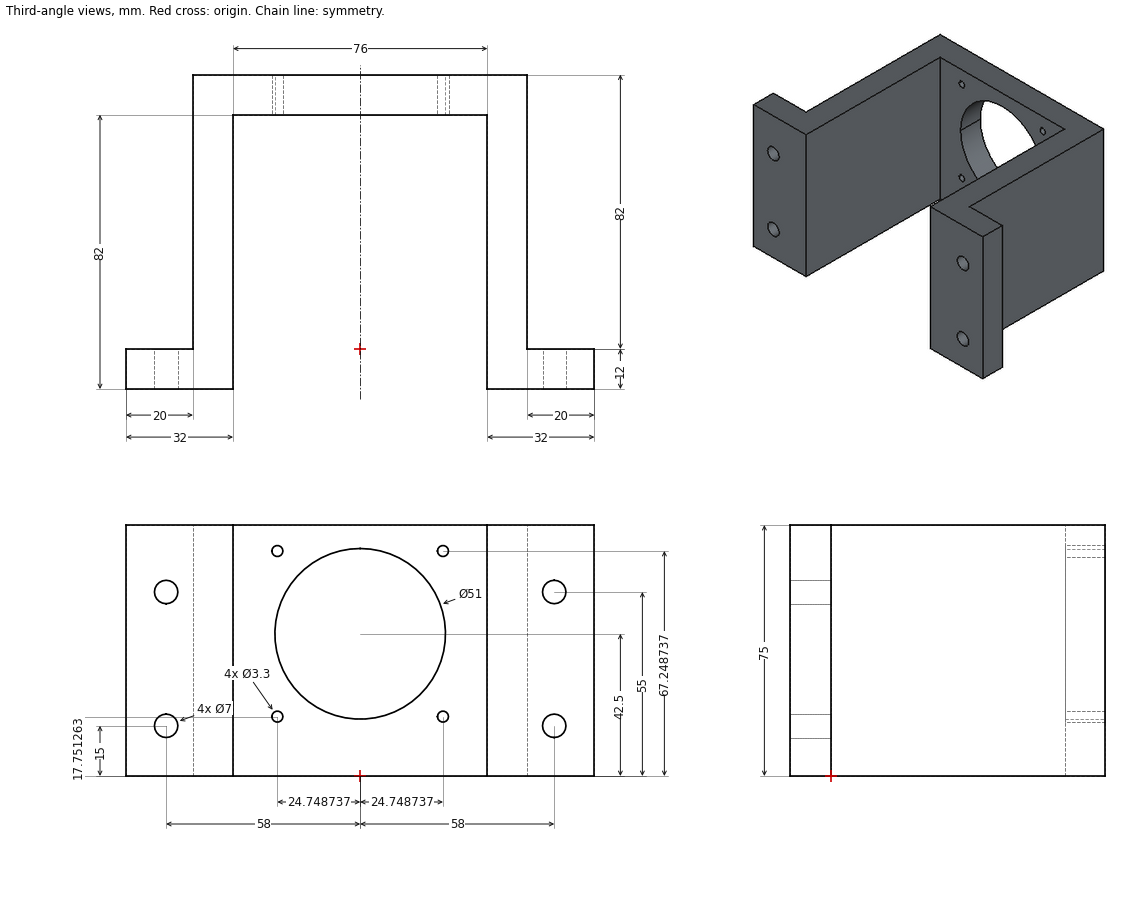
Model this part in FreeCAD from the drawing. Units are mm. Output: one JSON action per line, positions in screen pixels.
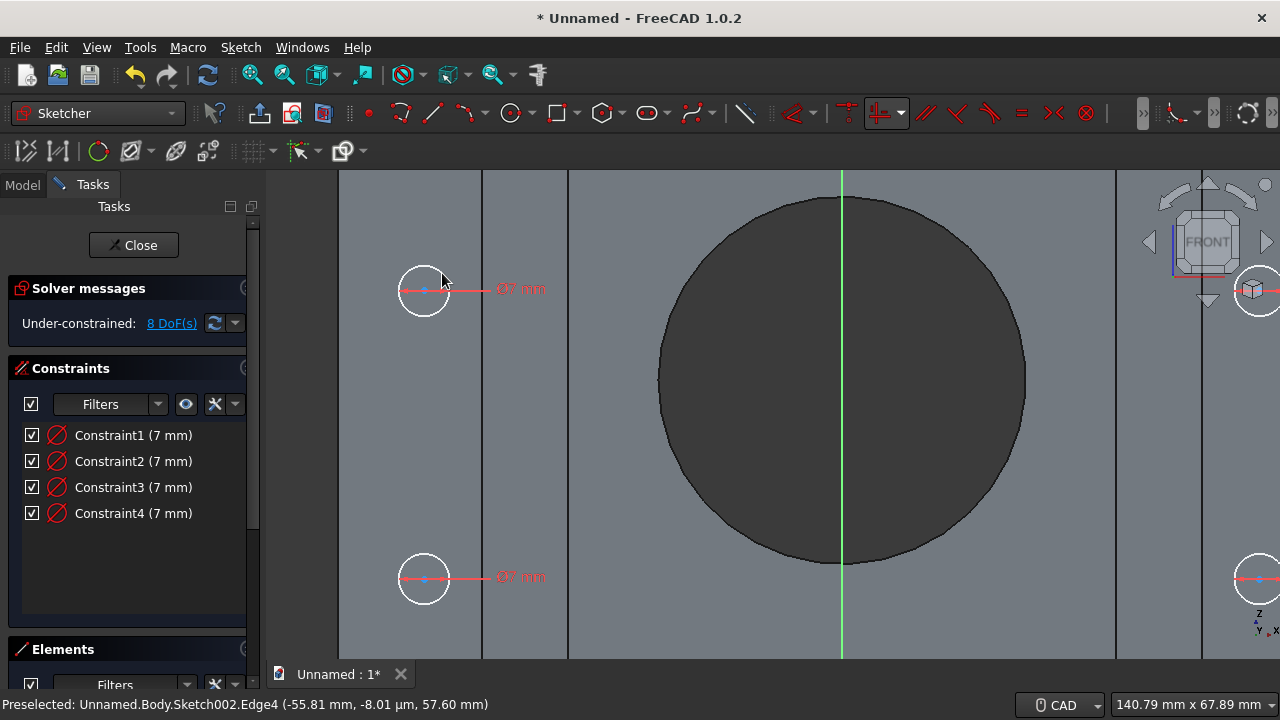
{"action": "left_click", "coordinate": [424, 579]}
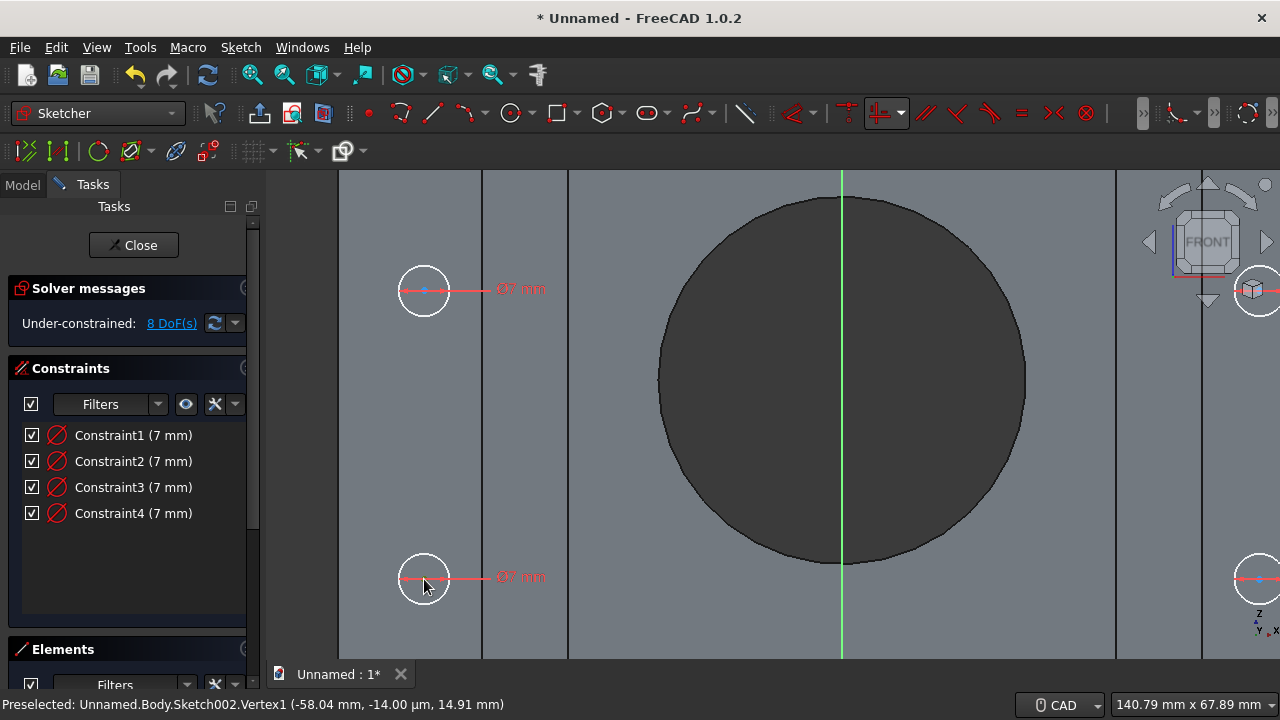
{"action": "scroll", "coordinate": [425, 290], "scroll_direction": "down", "scroll_amount": 2}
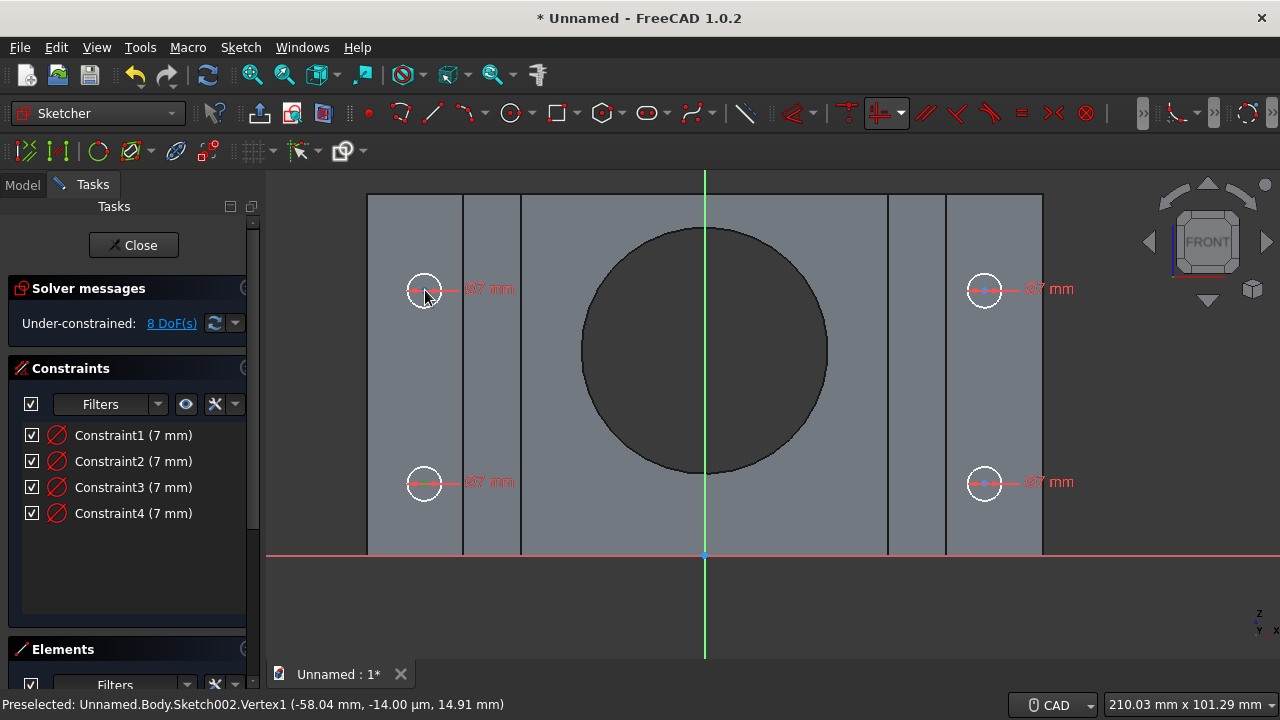
{"action": "left_click", "coordinate": [985, 484]}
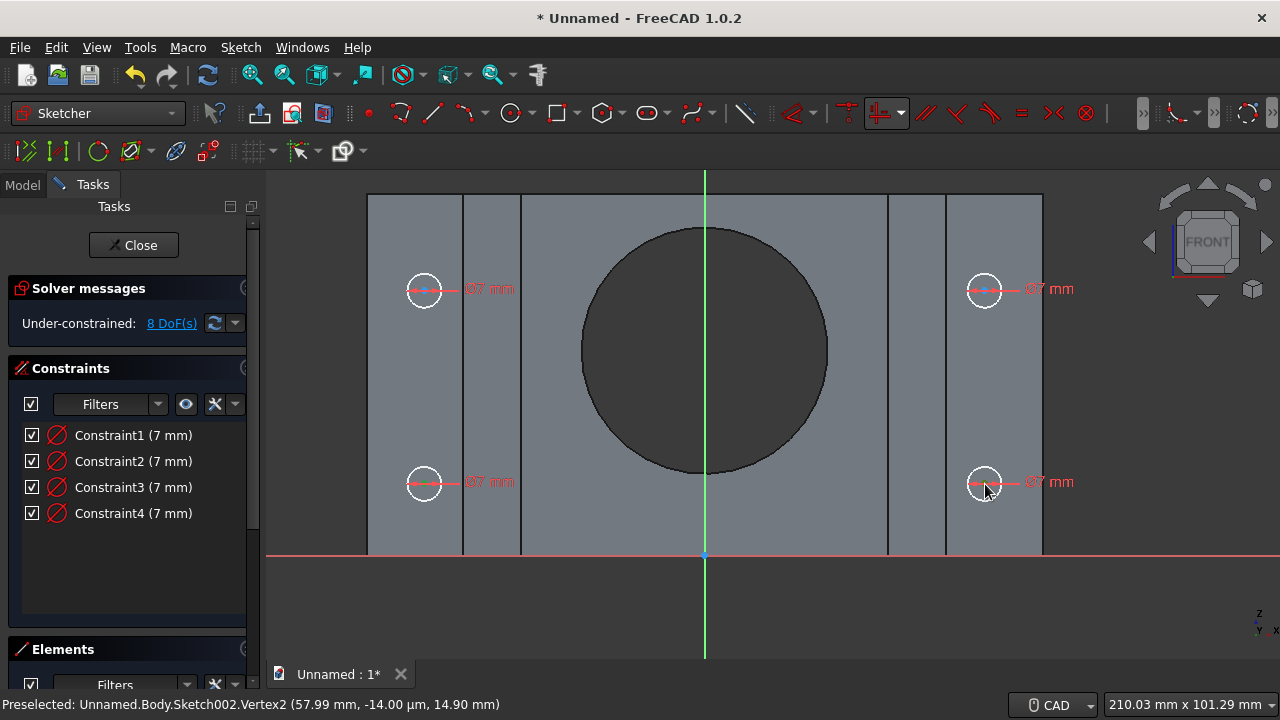
{"action": "key", "text": "h"}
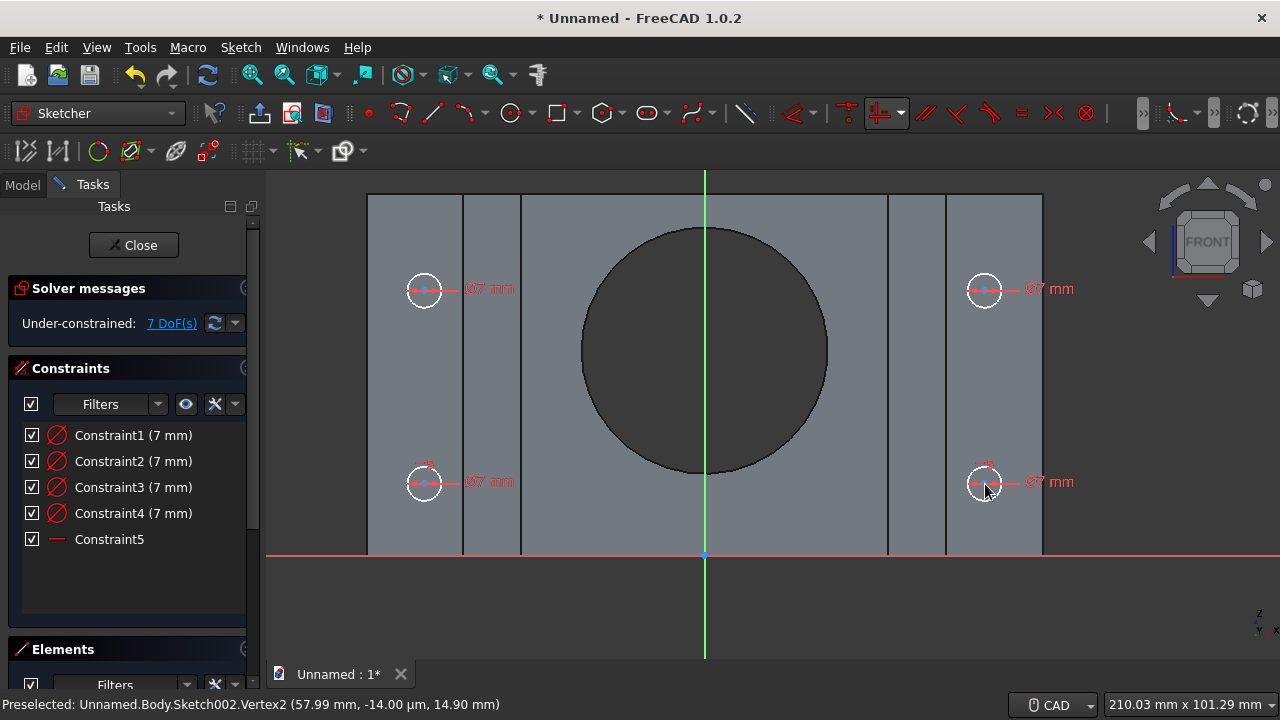
{"action": "left_click", "coordinate": [985, 484]}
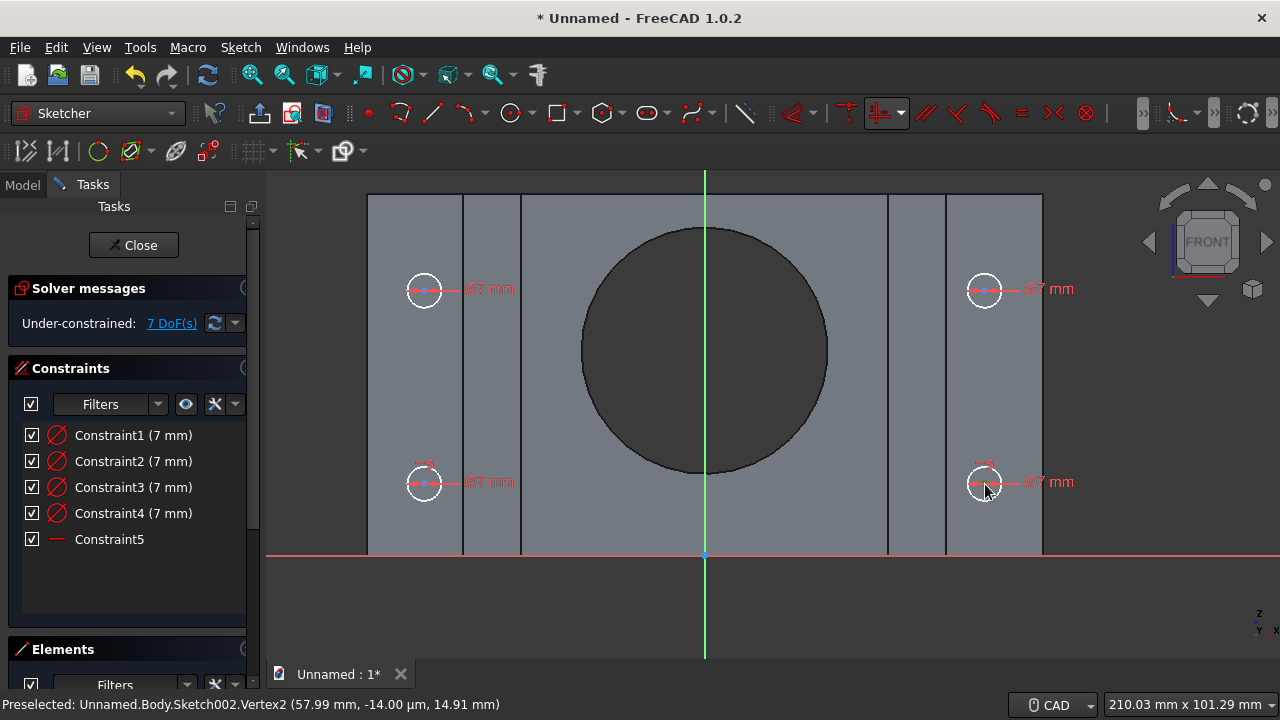
{"action": "left_click", "coordinate": [985, 291]}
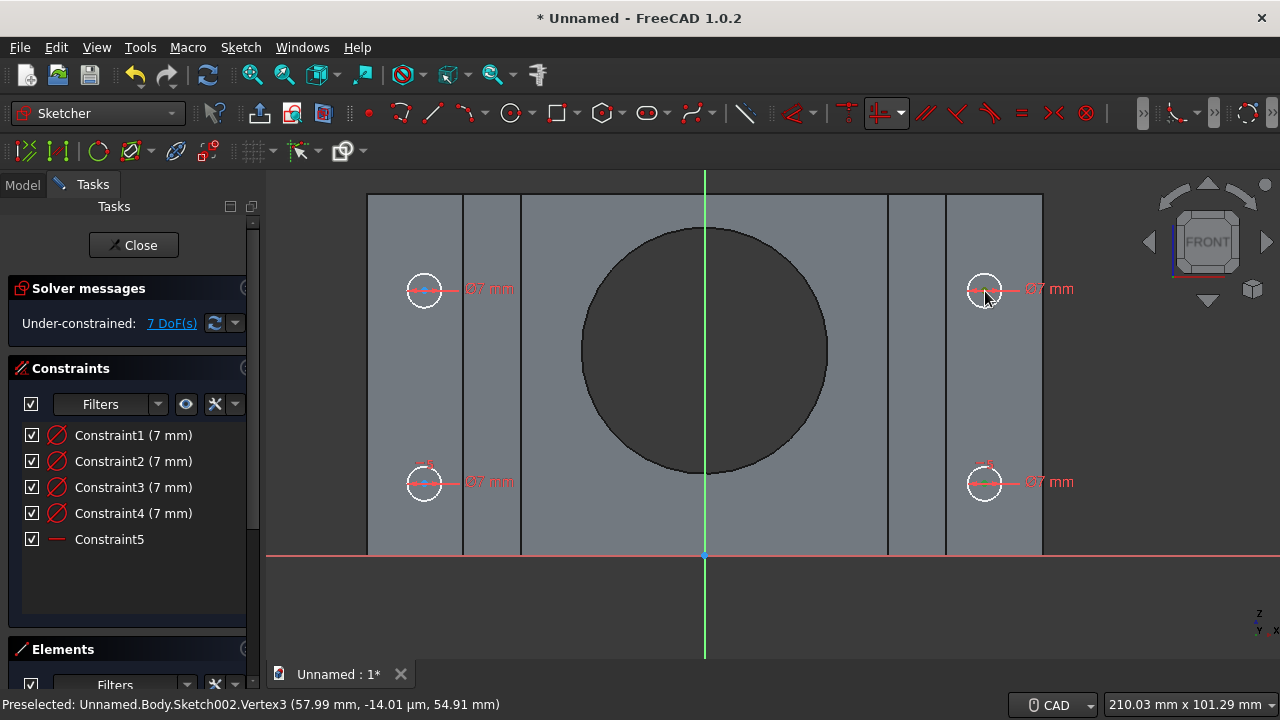
{"action": "key", "text": "v"}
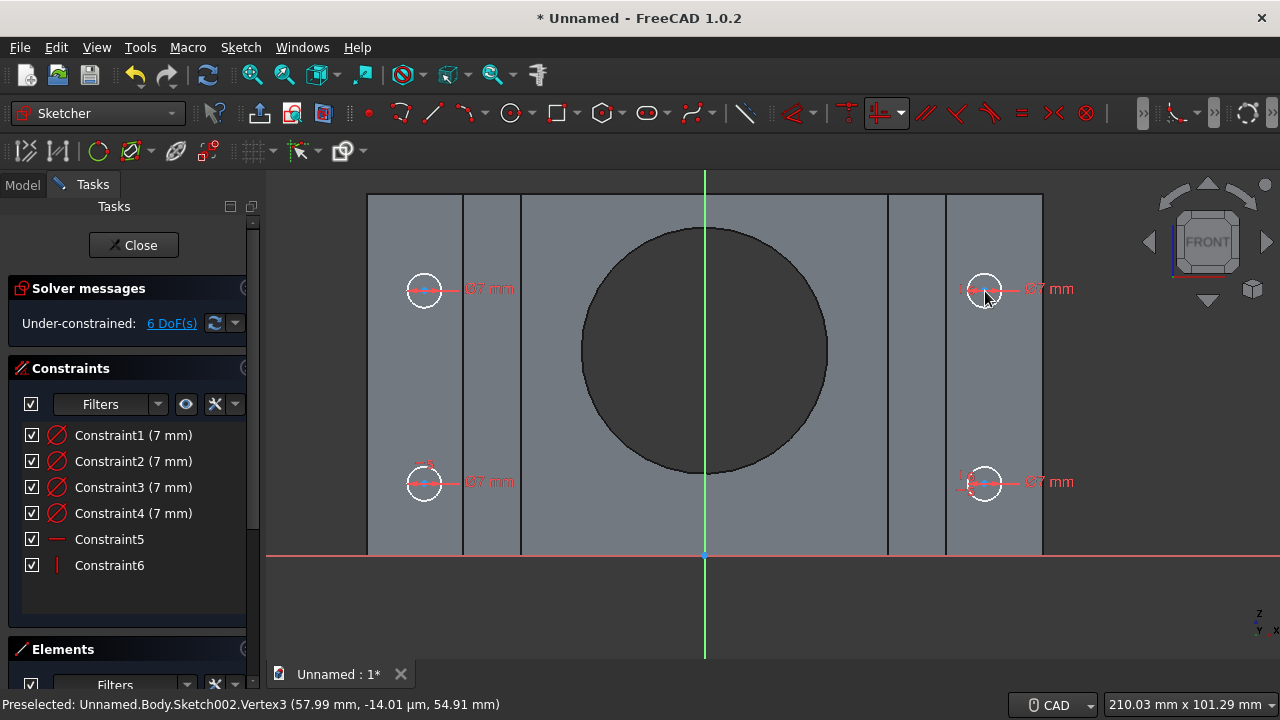
{"action": "left_click", "coordinate": [424, 484]}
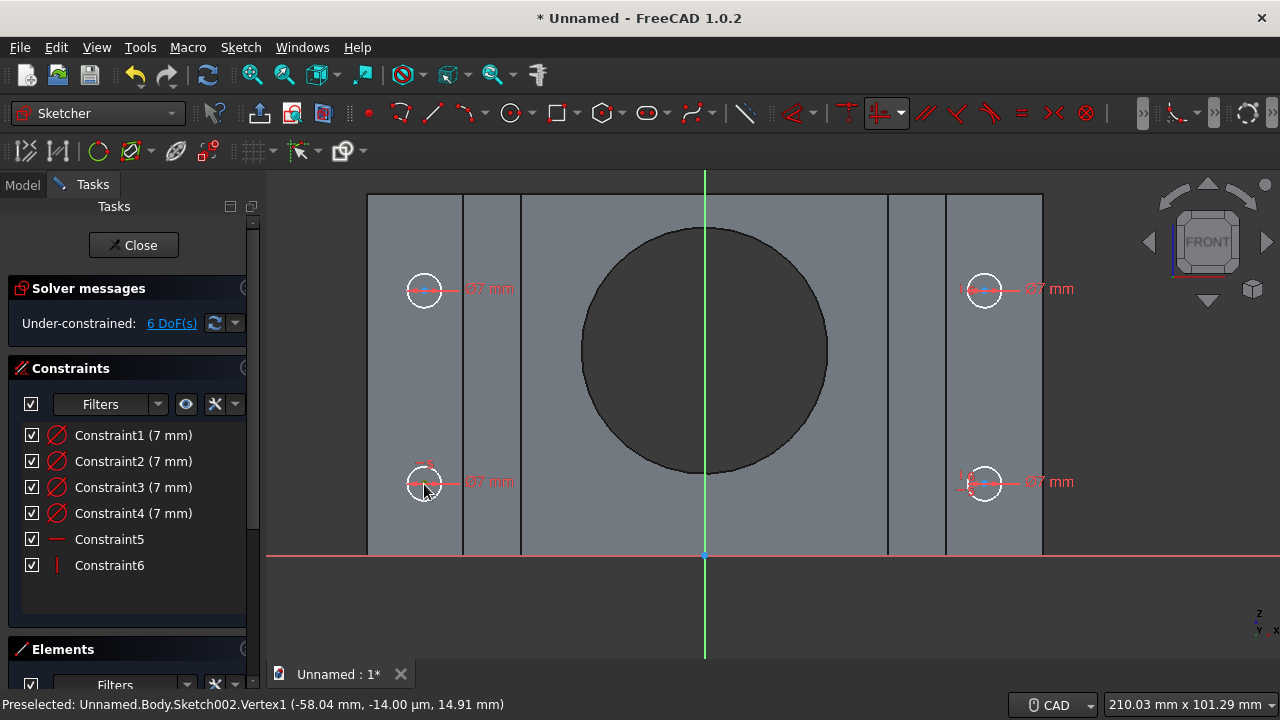
{"action": "left_click", "coordinate": [424, 291]}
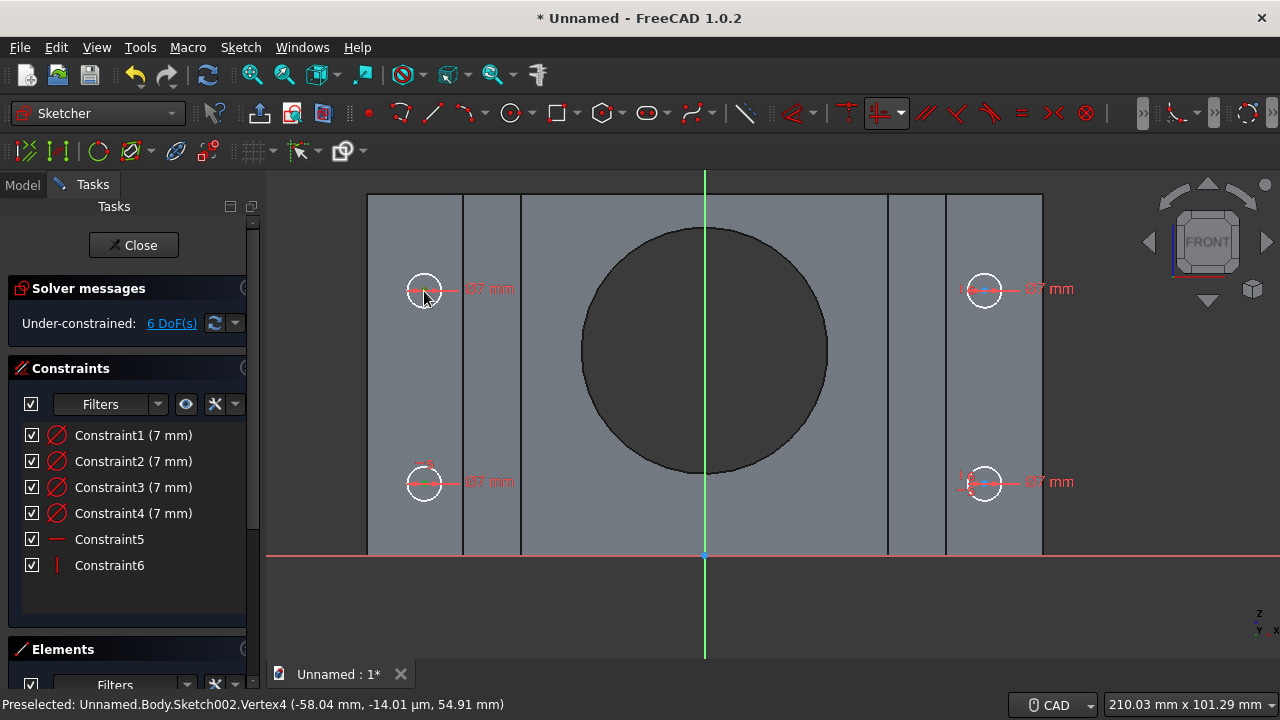
{"action": "left_click", "coordinate": [904, 114]}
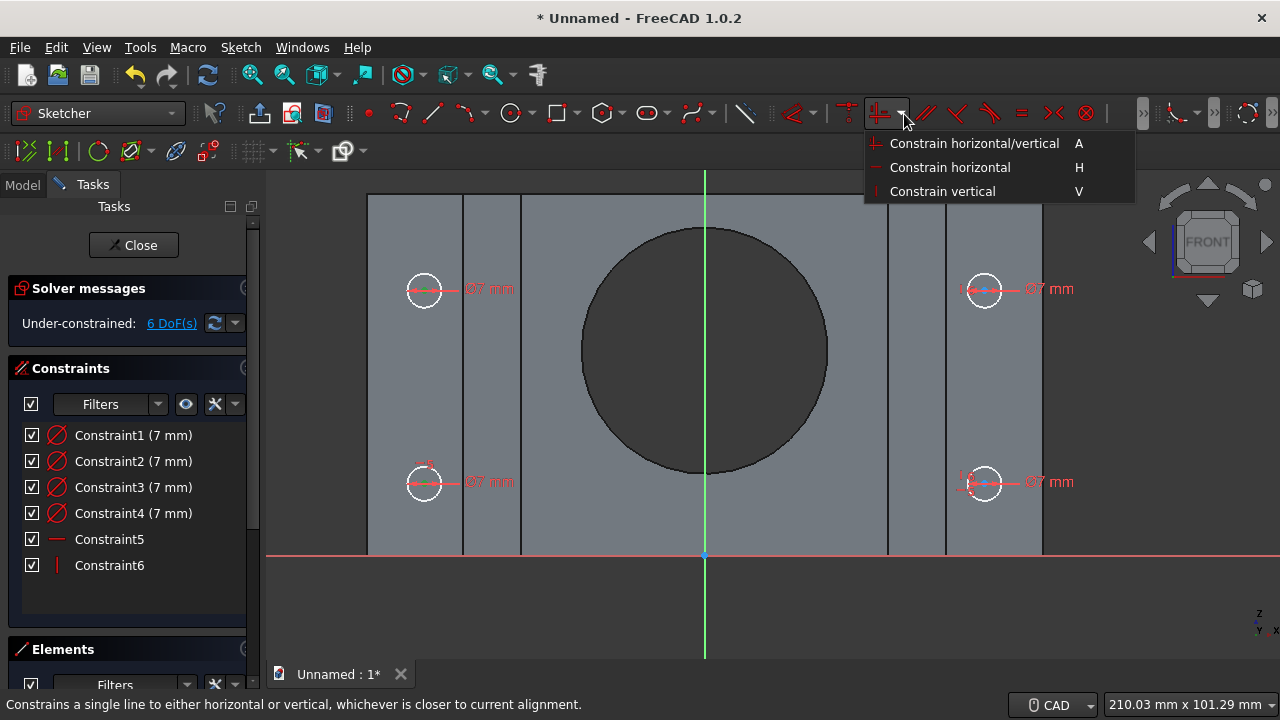
{"action": "left_click", "coordinate": [1000, 191]}